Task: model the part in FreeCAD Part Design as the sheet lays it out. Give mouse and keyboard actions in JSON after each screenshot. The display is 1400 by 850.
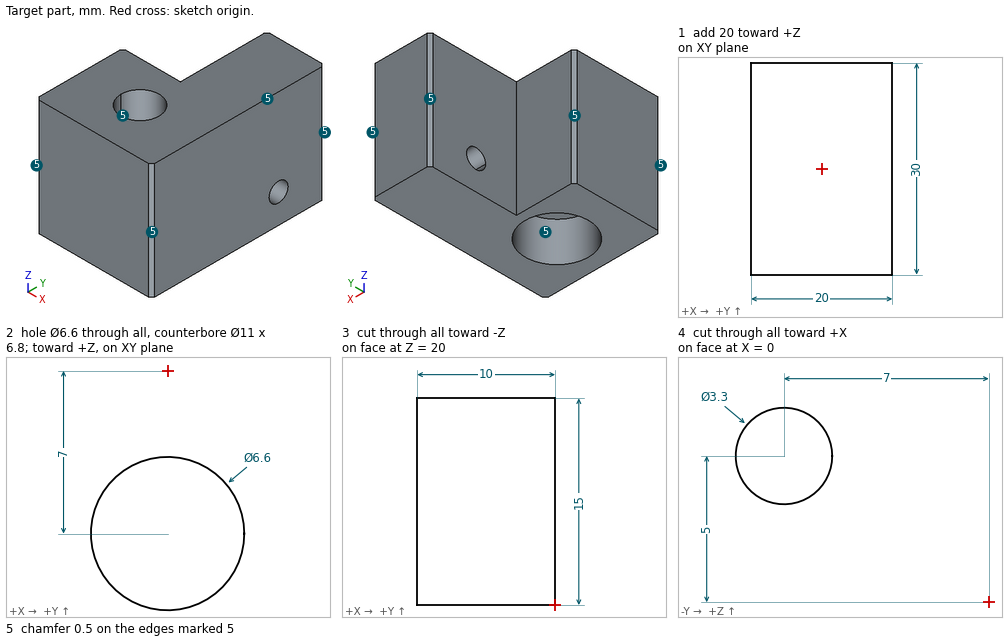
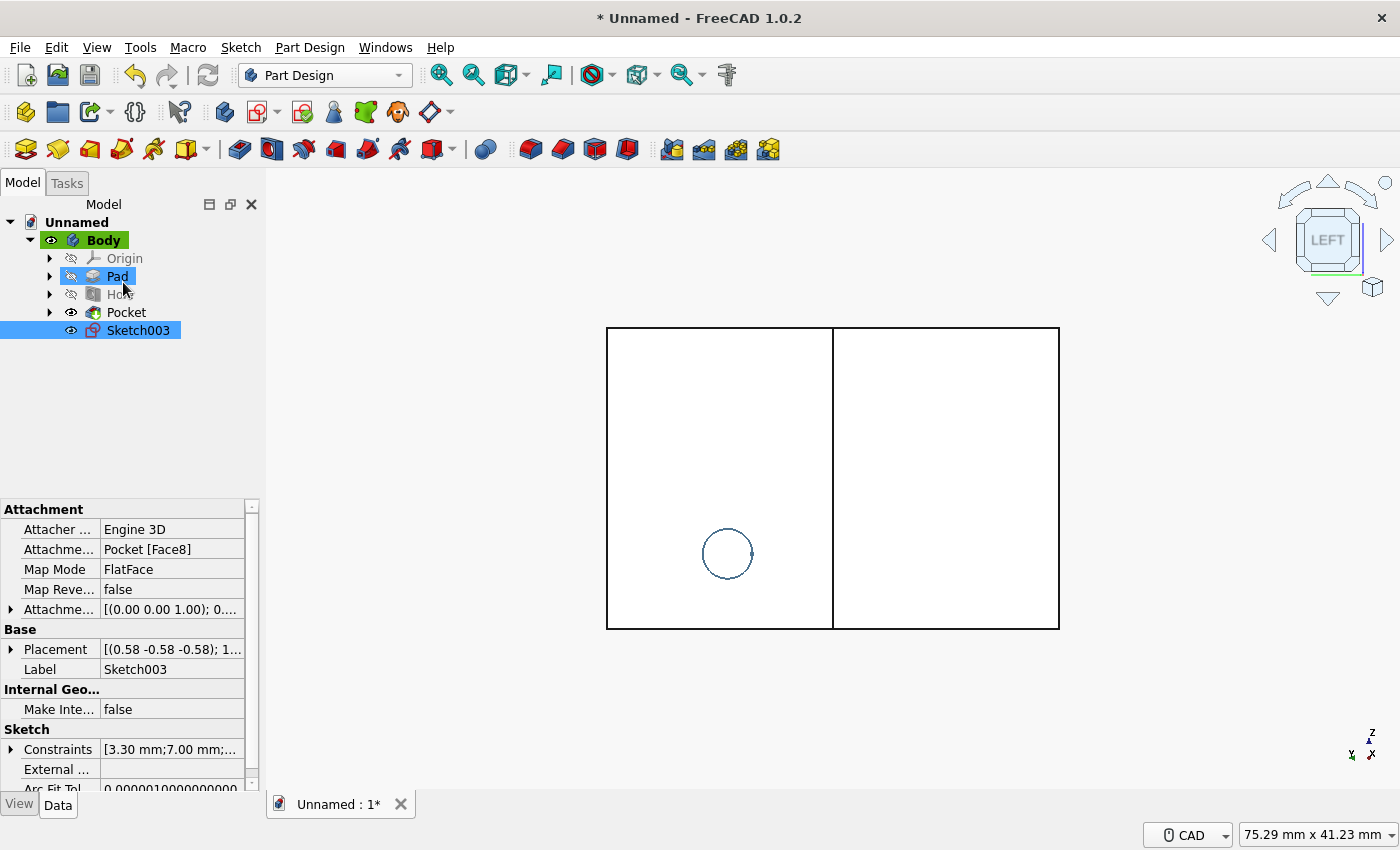
{"action": "left_click", "coordinate": [240, 150]}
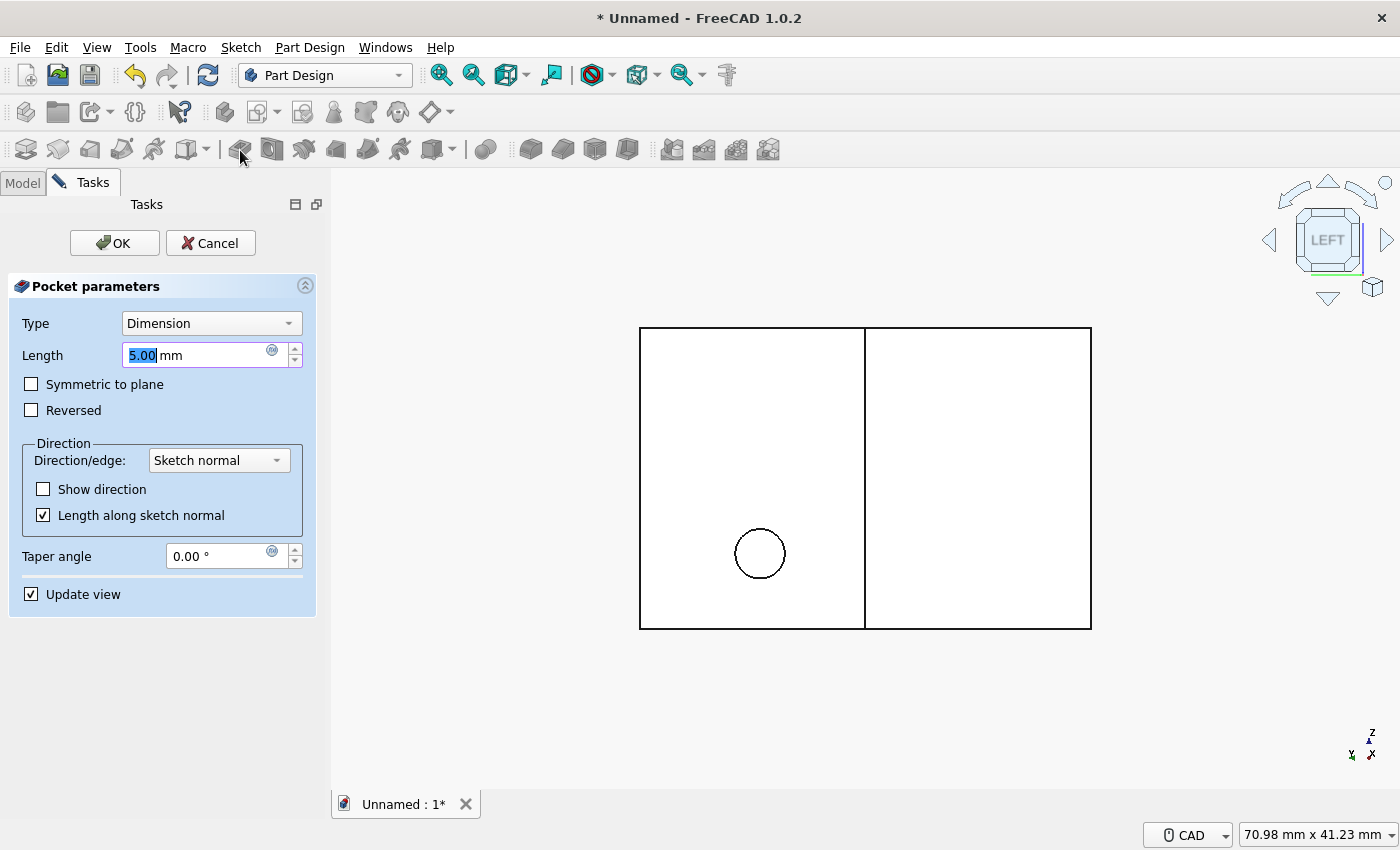
{"action": "left_click", "coordinate": [212, 324]}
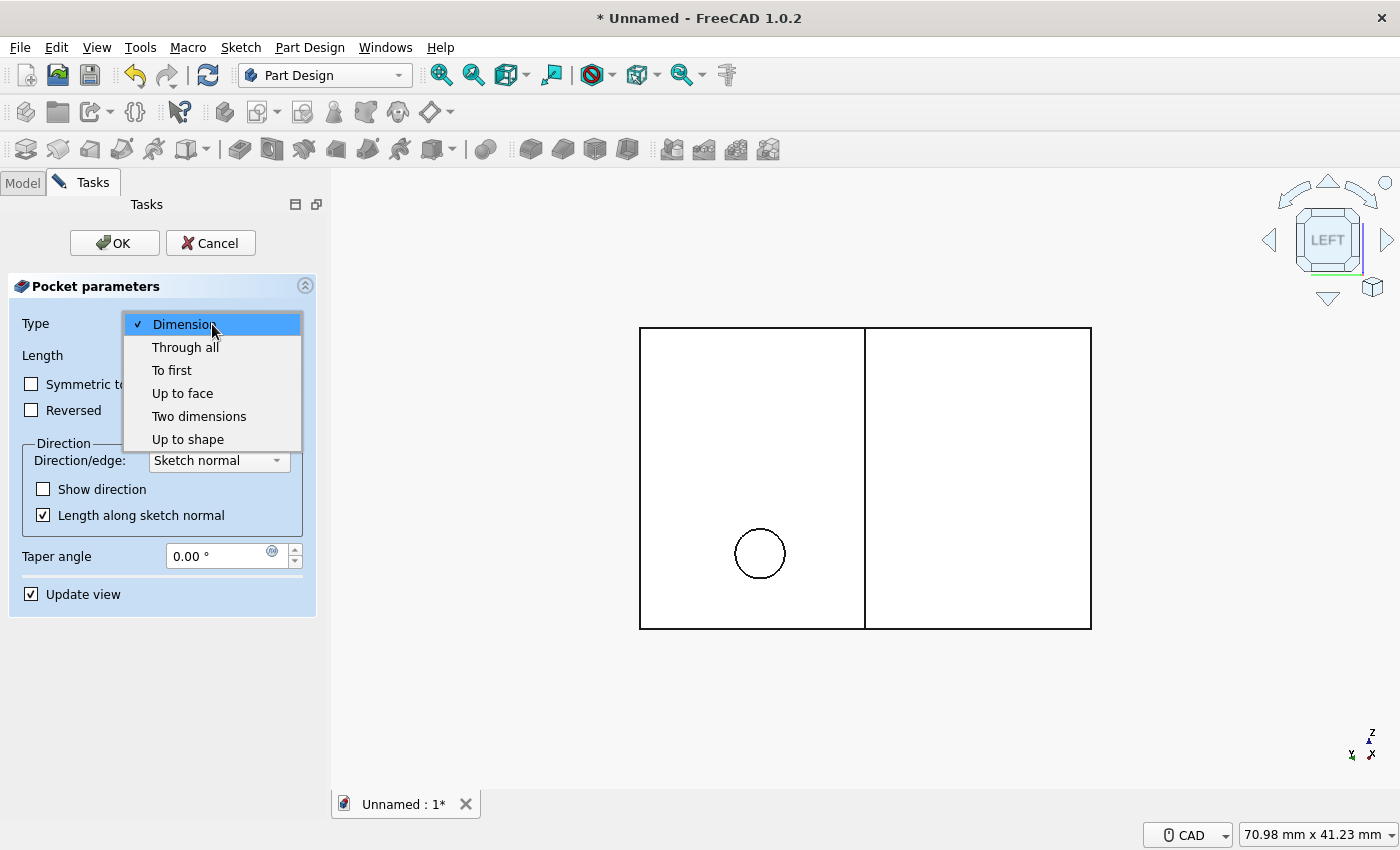
{"action": "left_click", "coordinate": [212, 348]}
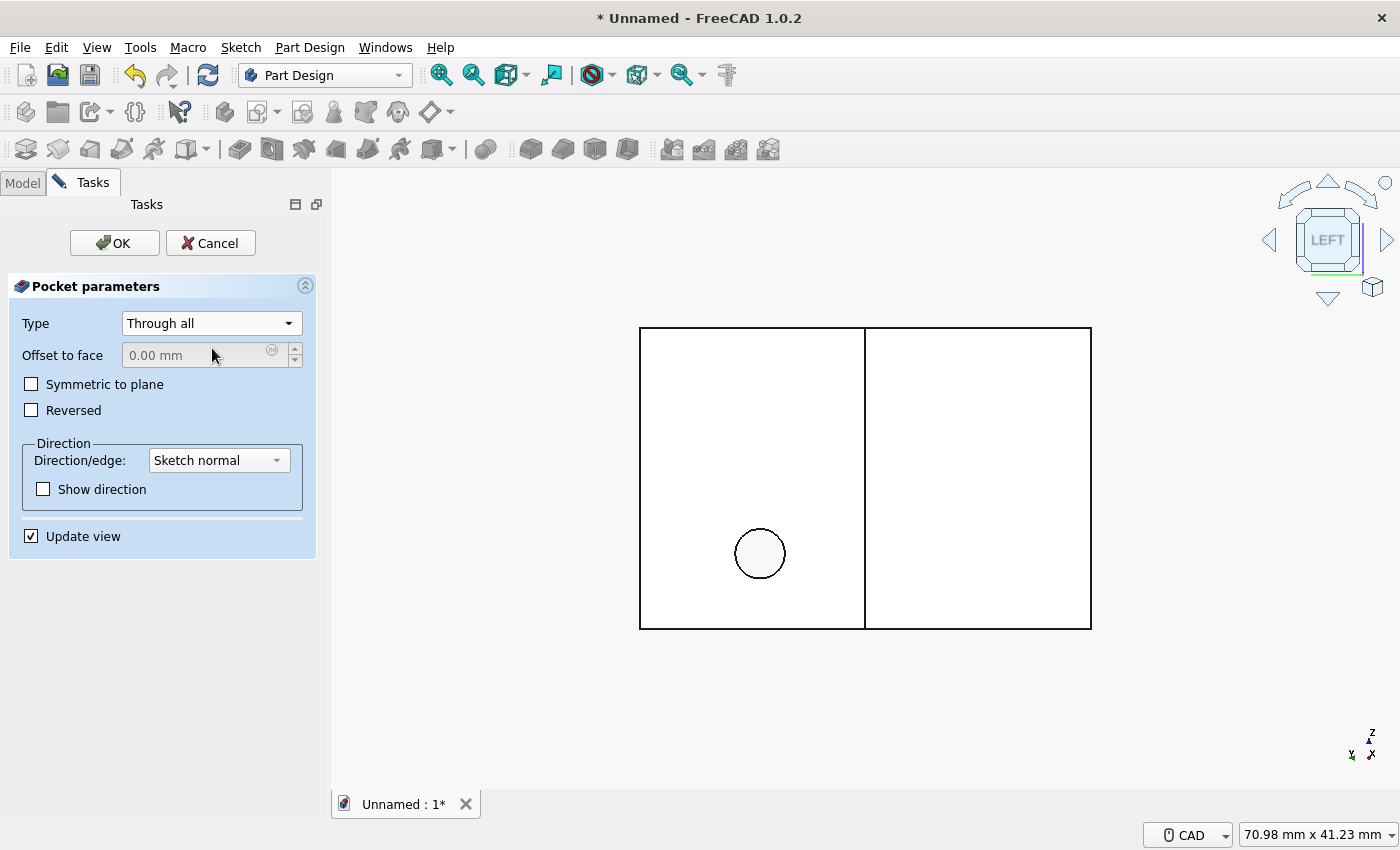
{"action": "left_click", "coordinate": [115, 243]}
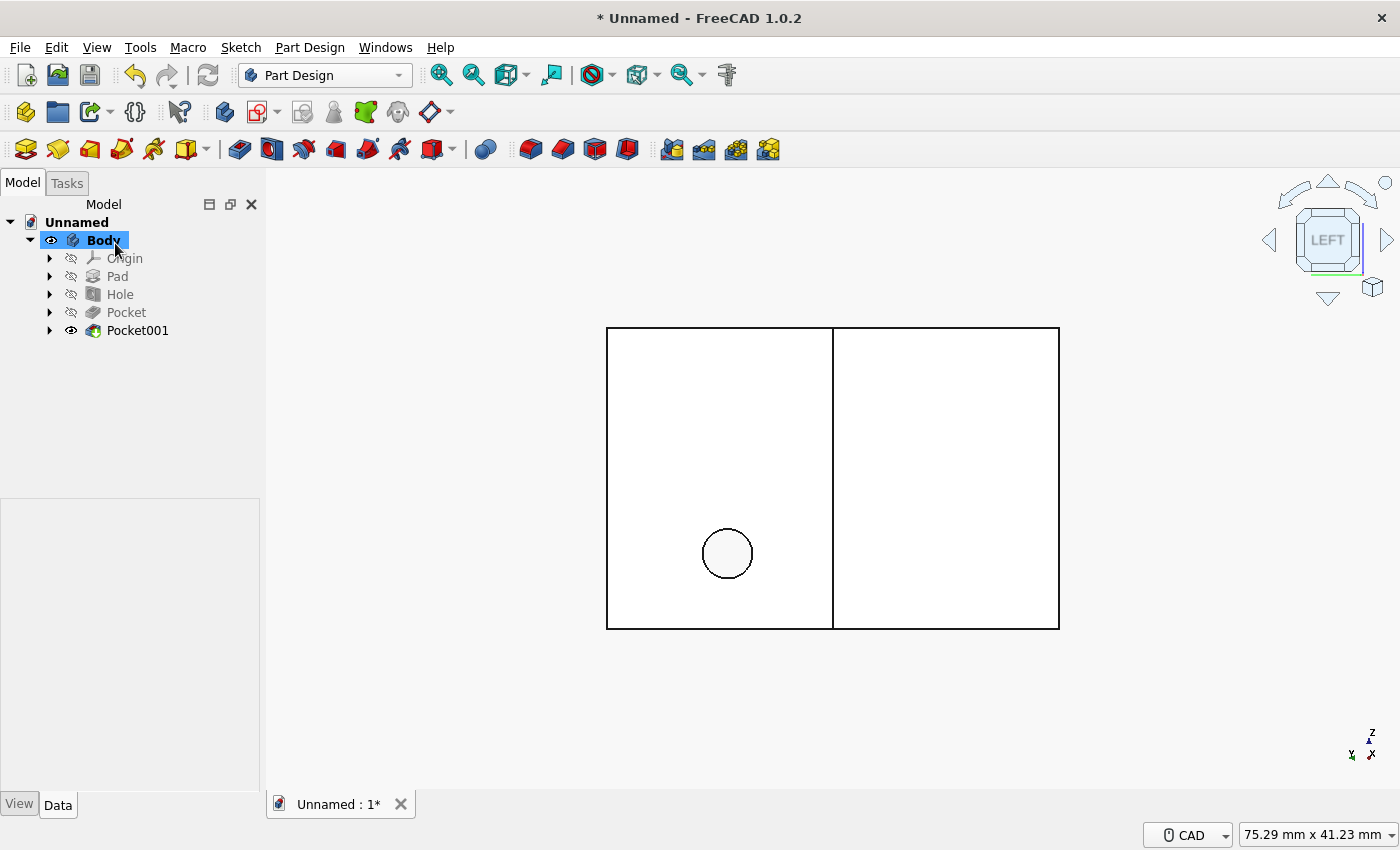
{"action": "left_click", "coordinate": [833, 477]}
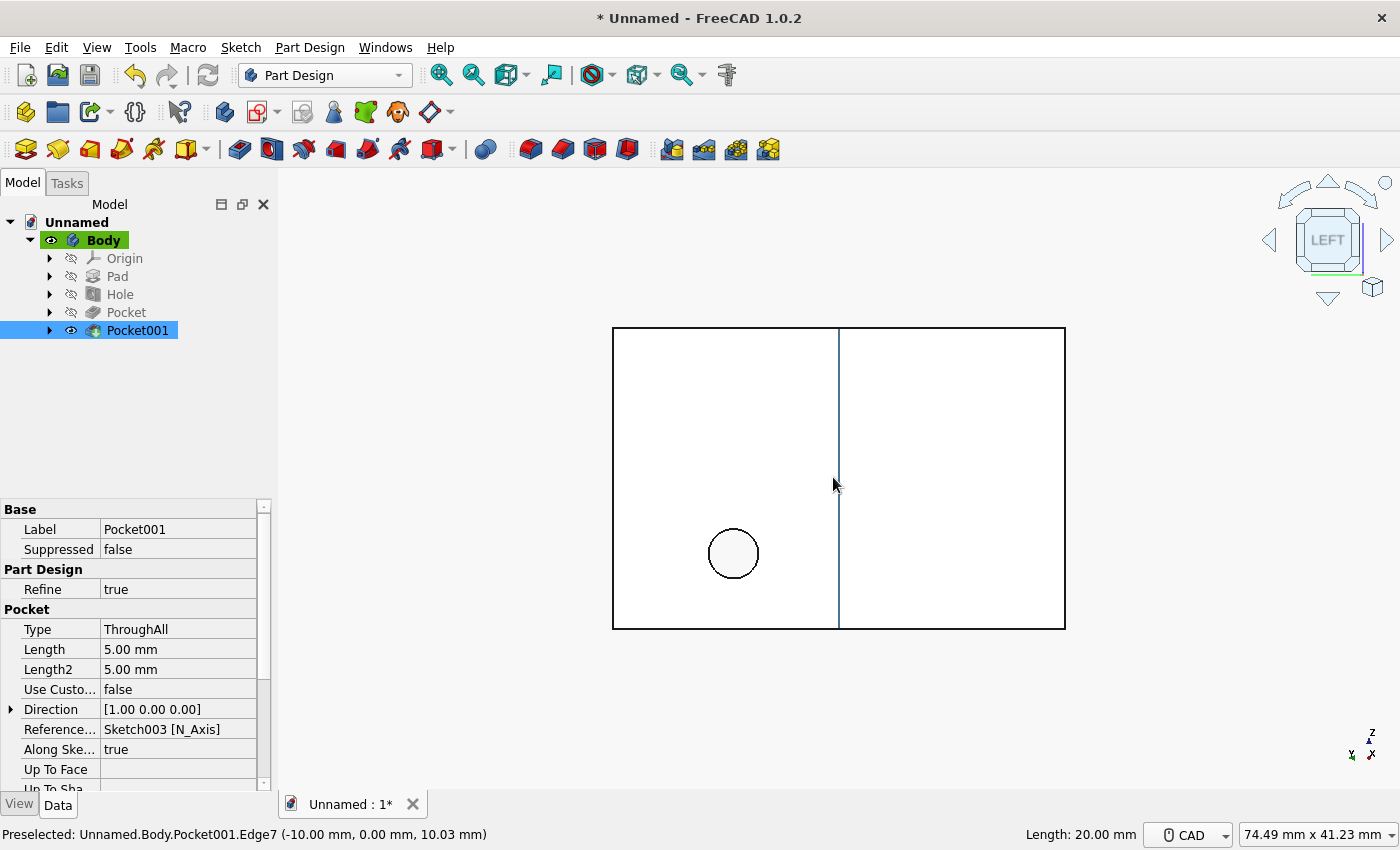
{"action": "left_click", "coordinate": [613, 477], "text": "ctrl"}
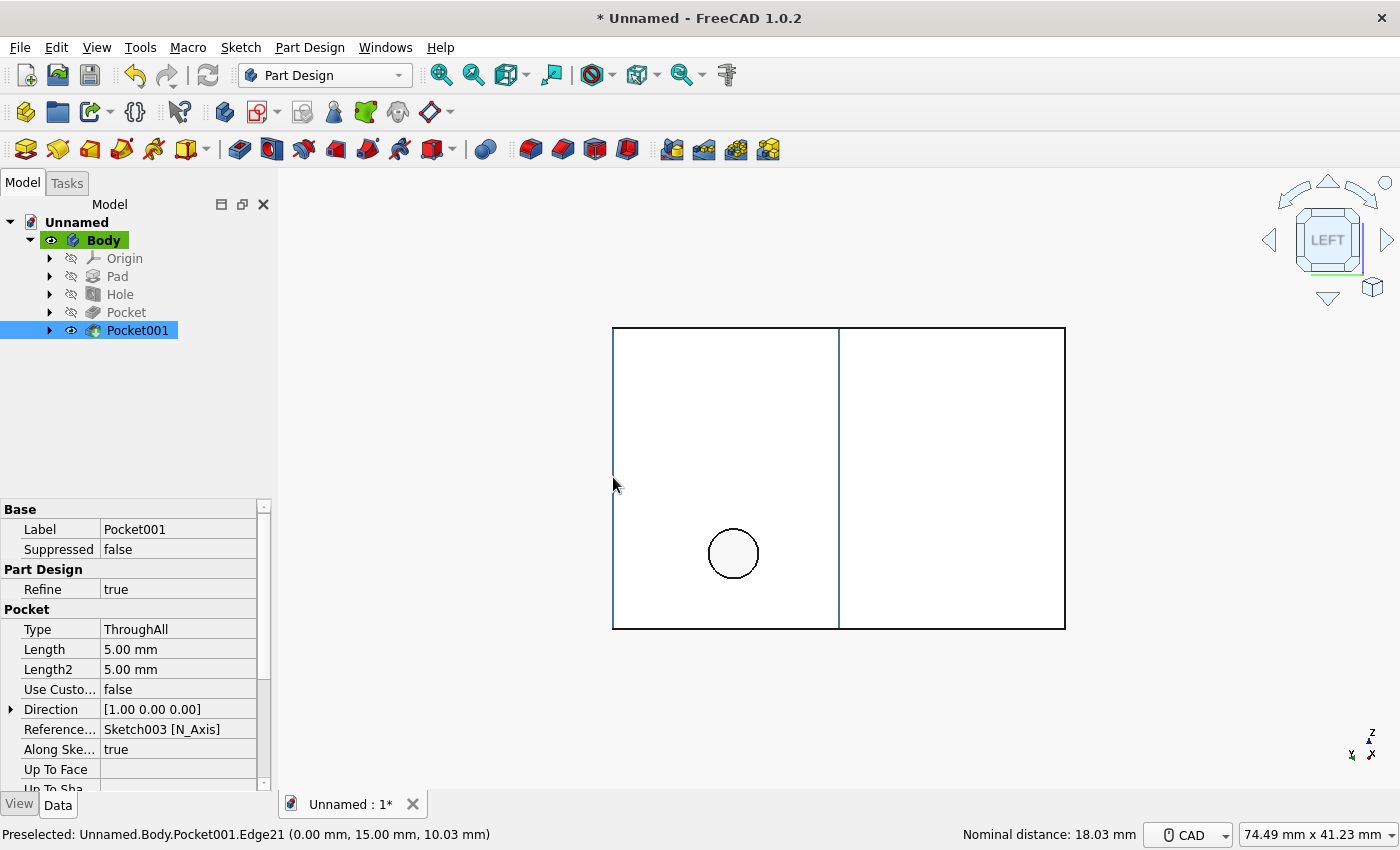
{"action": "left_click", "coordinate": [1065, 477], "text": "ctrl"}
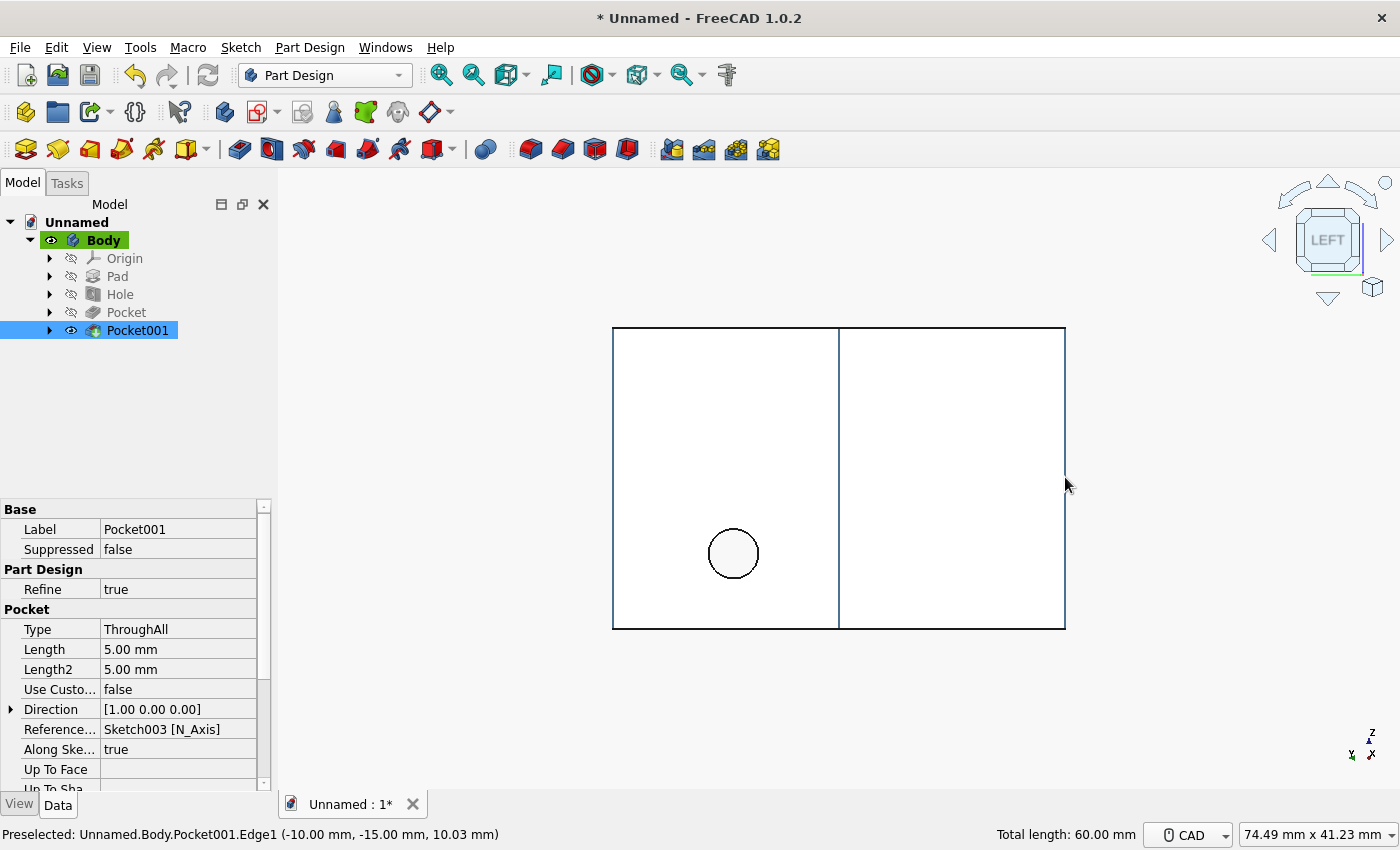
{"action": "key", "text": "0"}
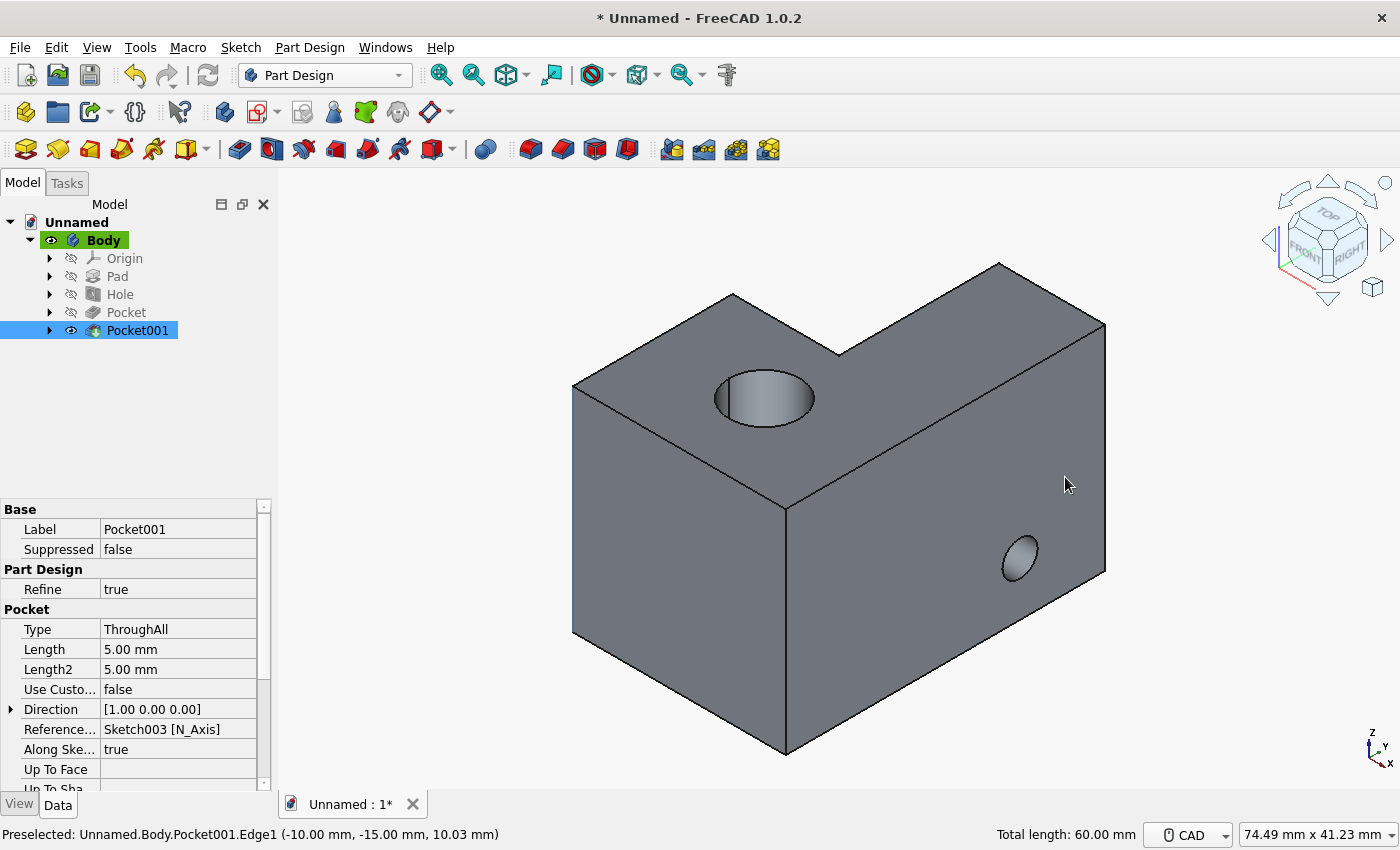
{"action": "left_click", "coordinate": [786, 631], "text": "ctrl"}